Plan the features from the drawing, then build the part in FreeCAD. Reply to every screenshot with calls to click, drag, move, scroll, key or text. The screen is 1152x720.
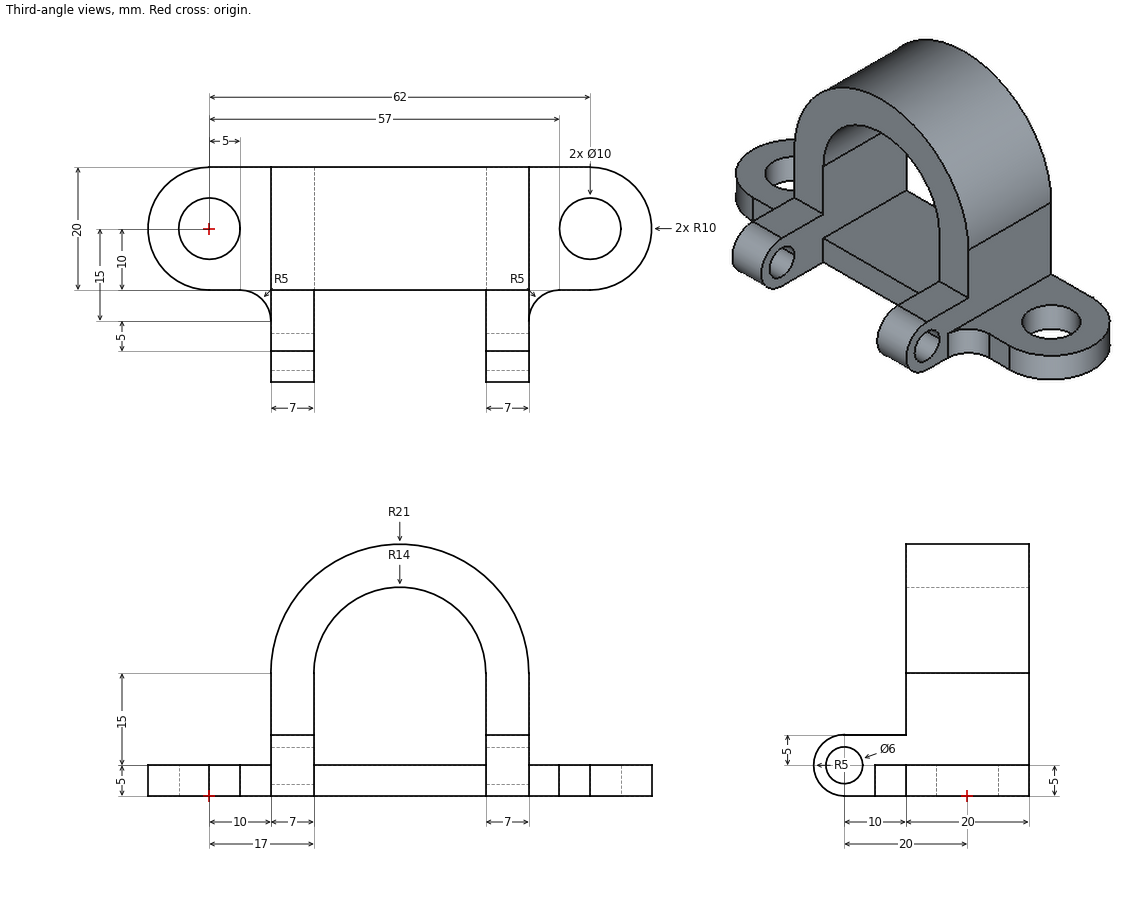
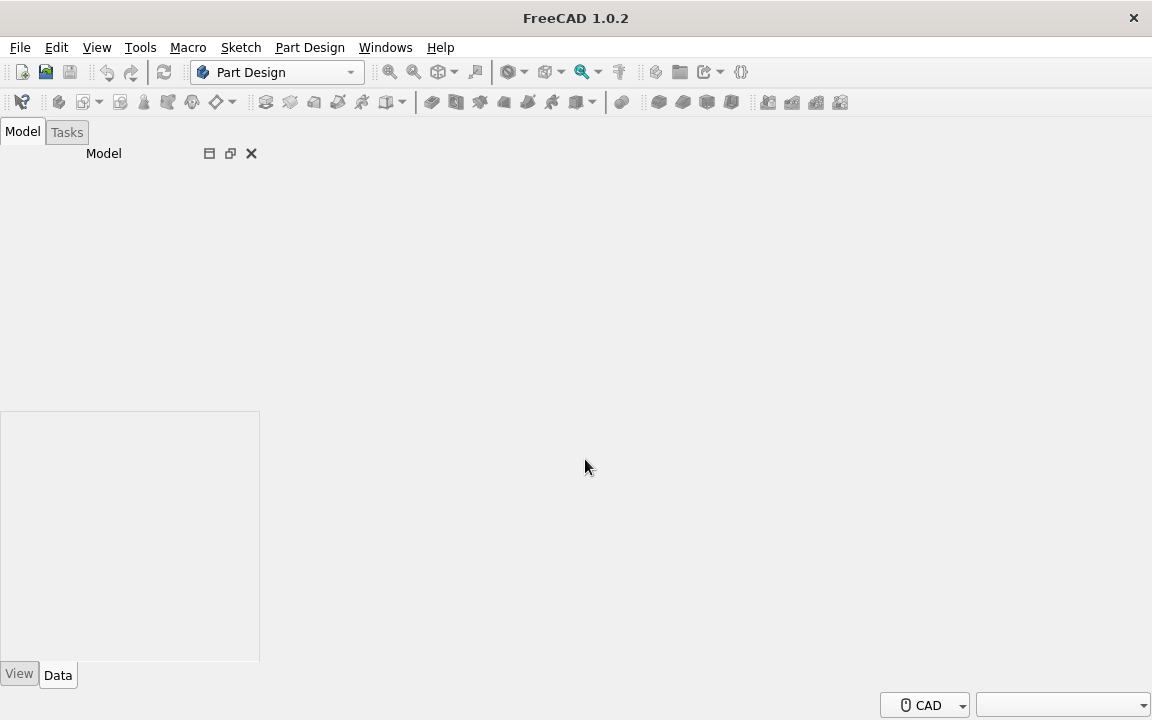
click(22, 72)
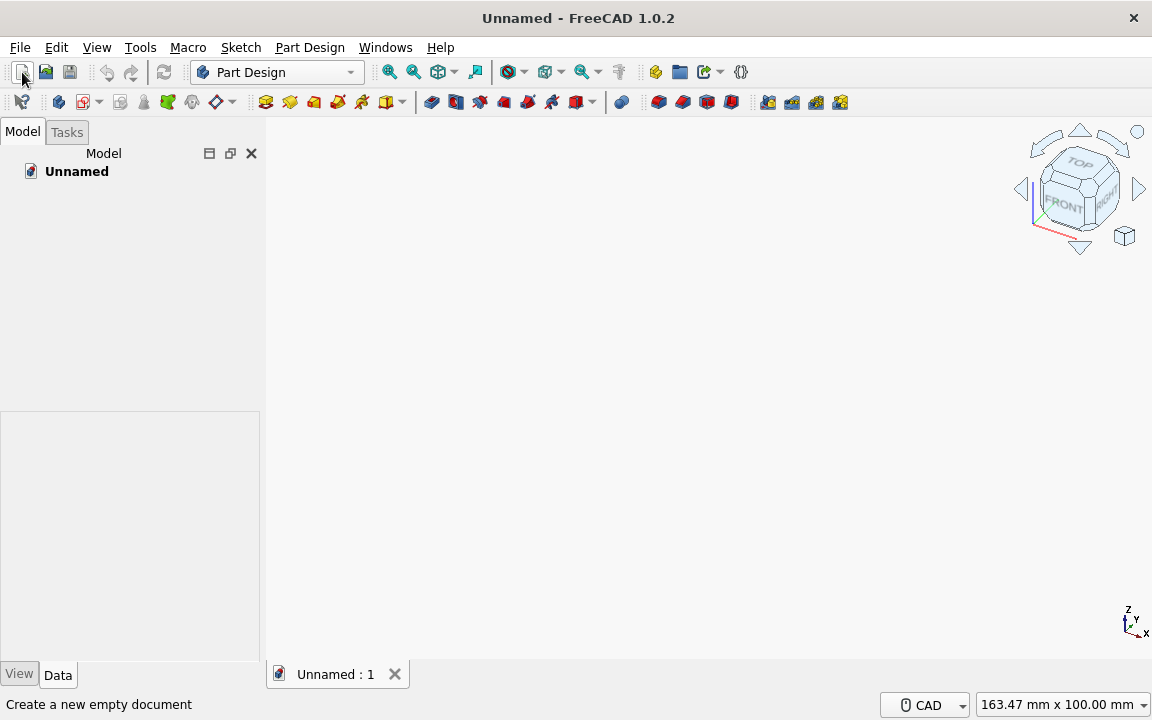
click(84, 102)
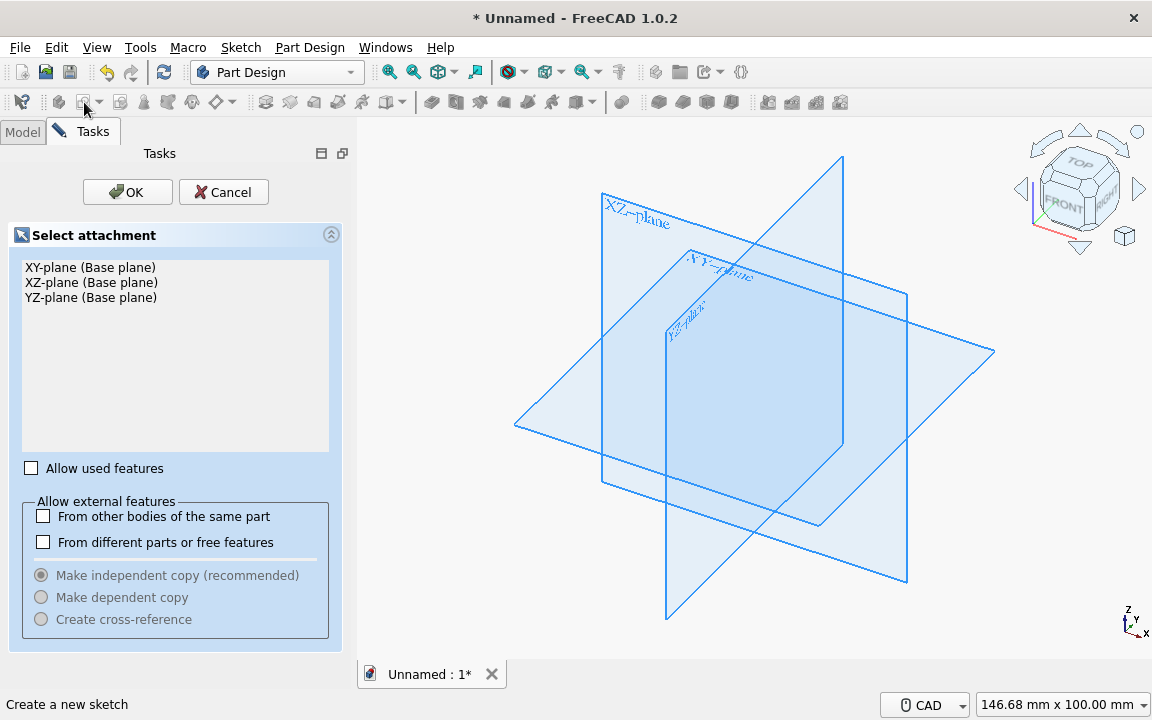
click(82, 268)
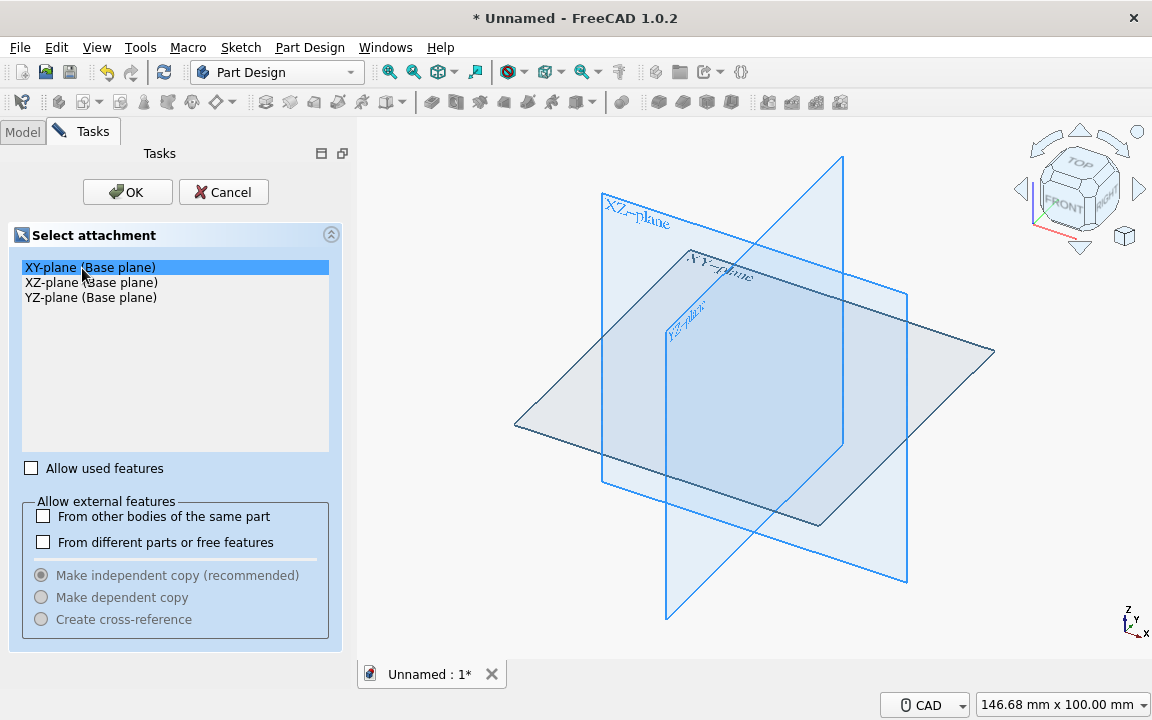
click(128, 192)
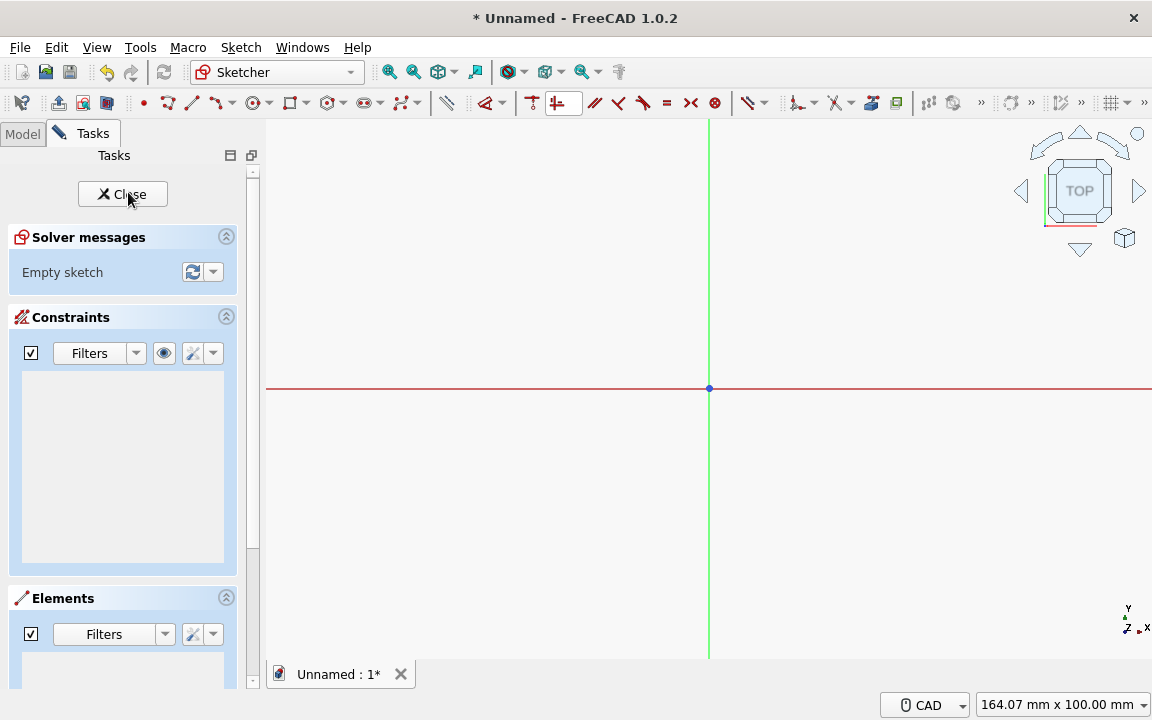
scroll(294, 389, down, 1)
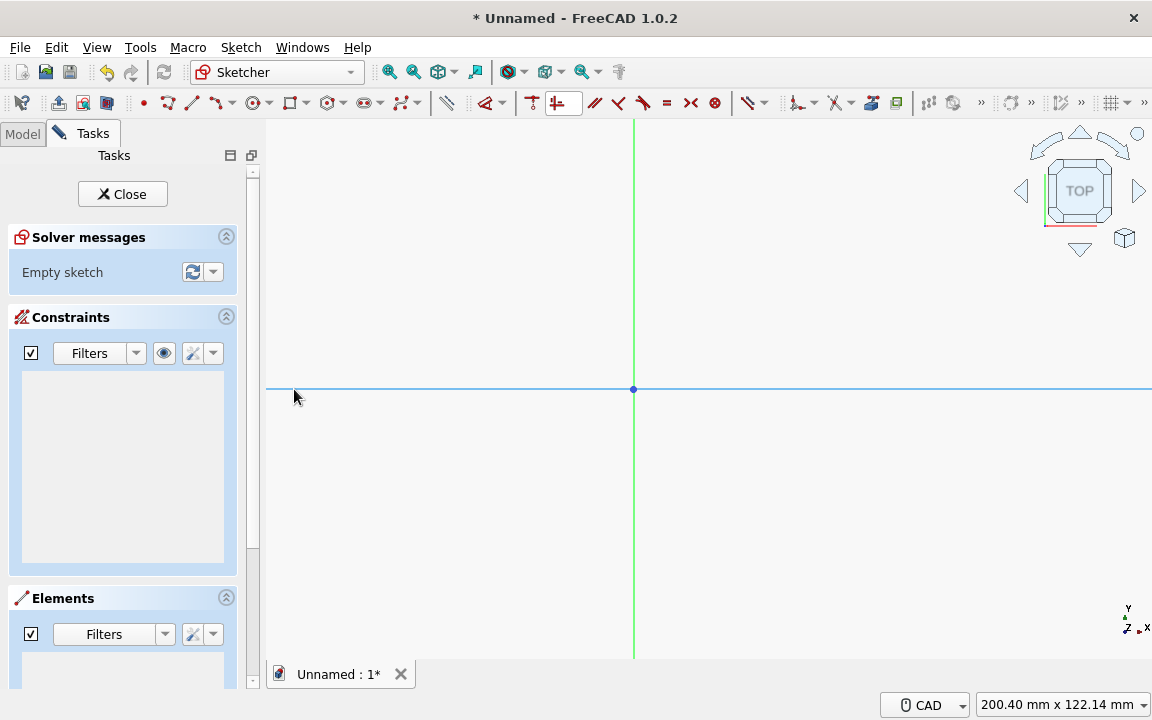
click(364, 104)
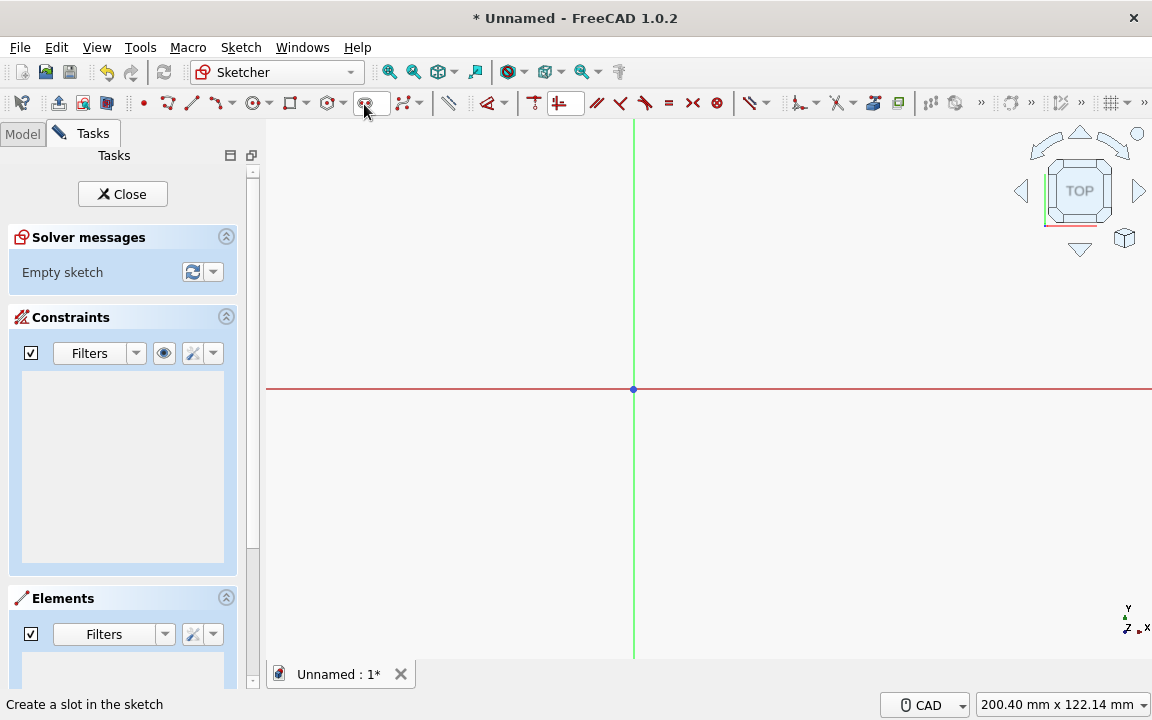
click(634, 389)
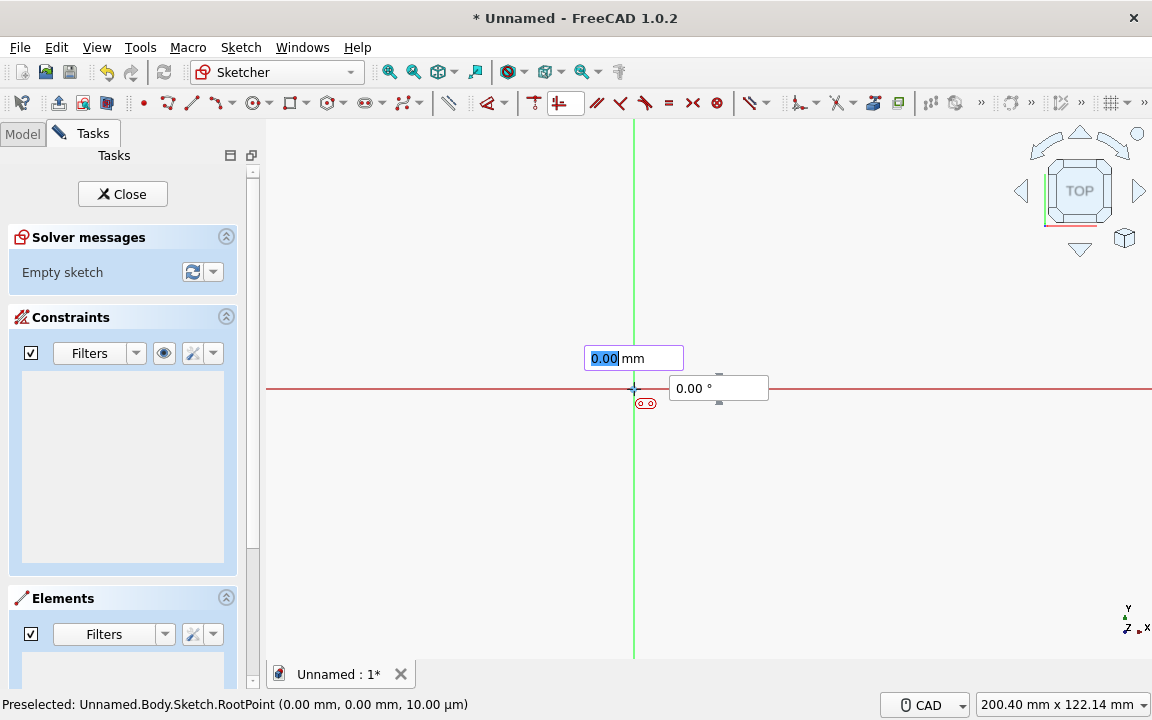
click(908, 380)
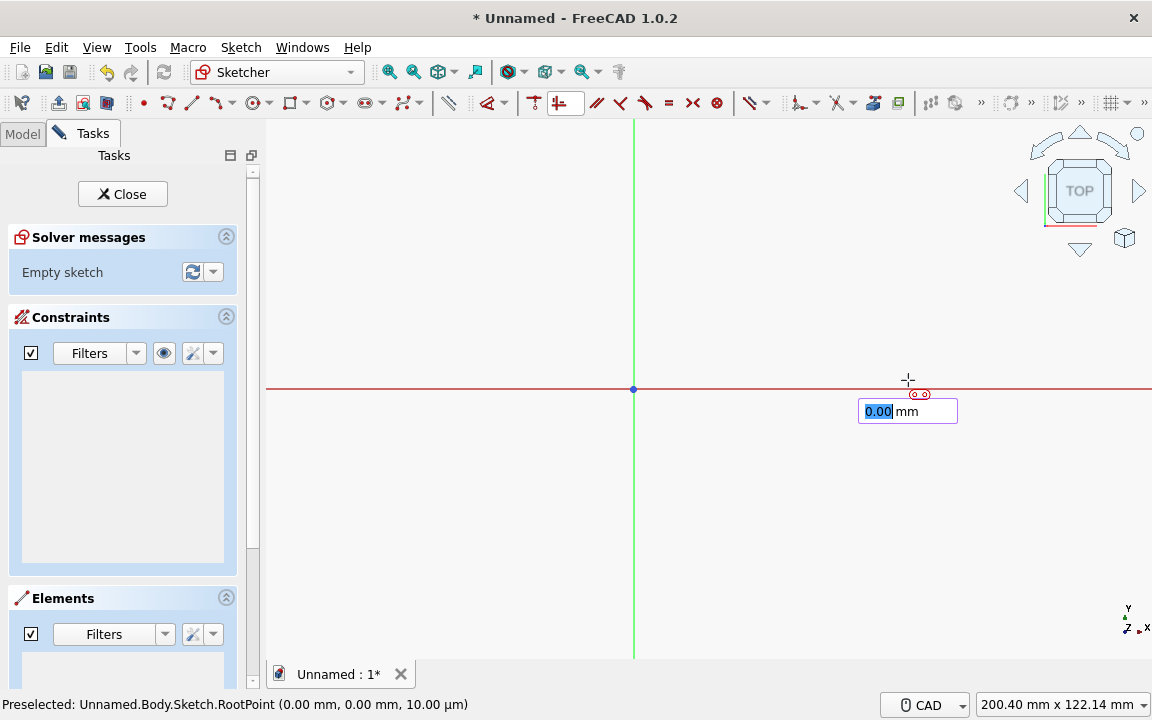
click(771, 433)
key(Escape)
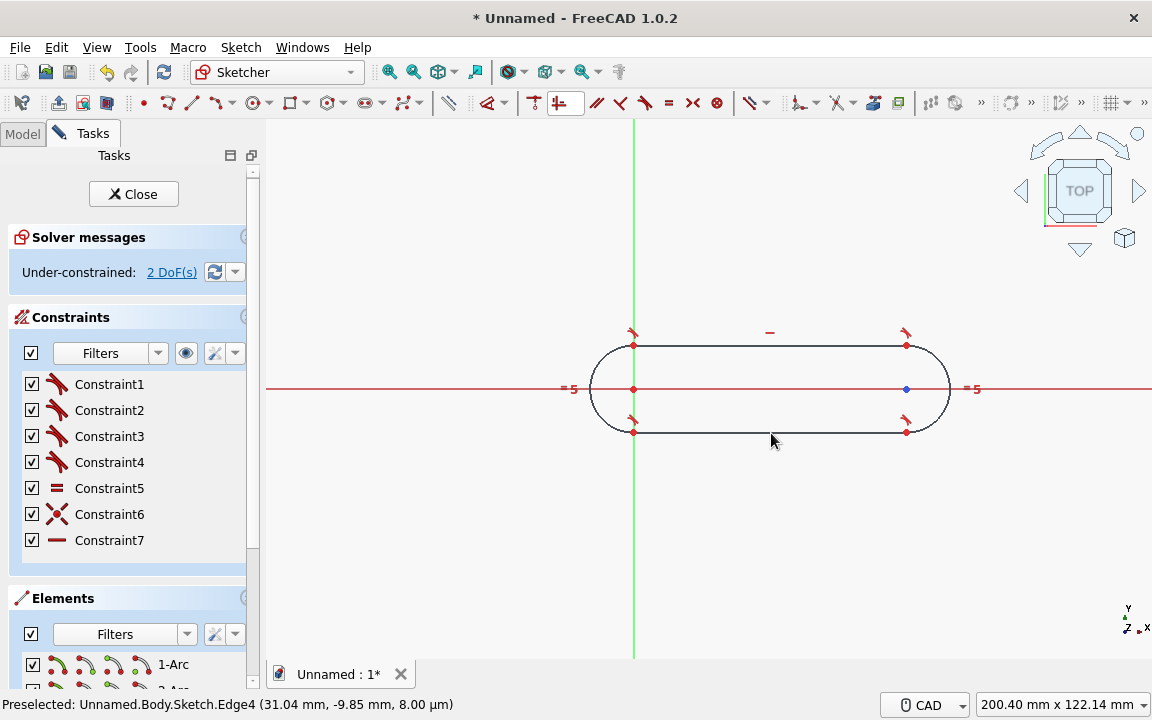
click(488, 104)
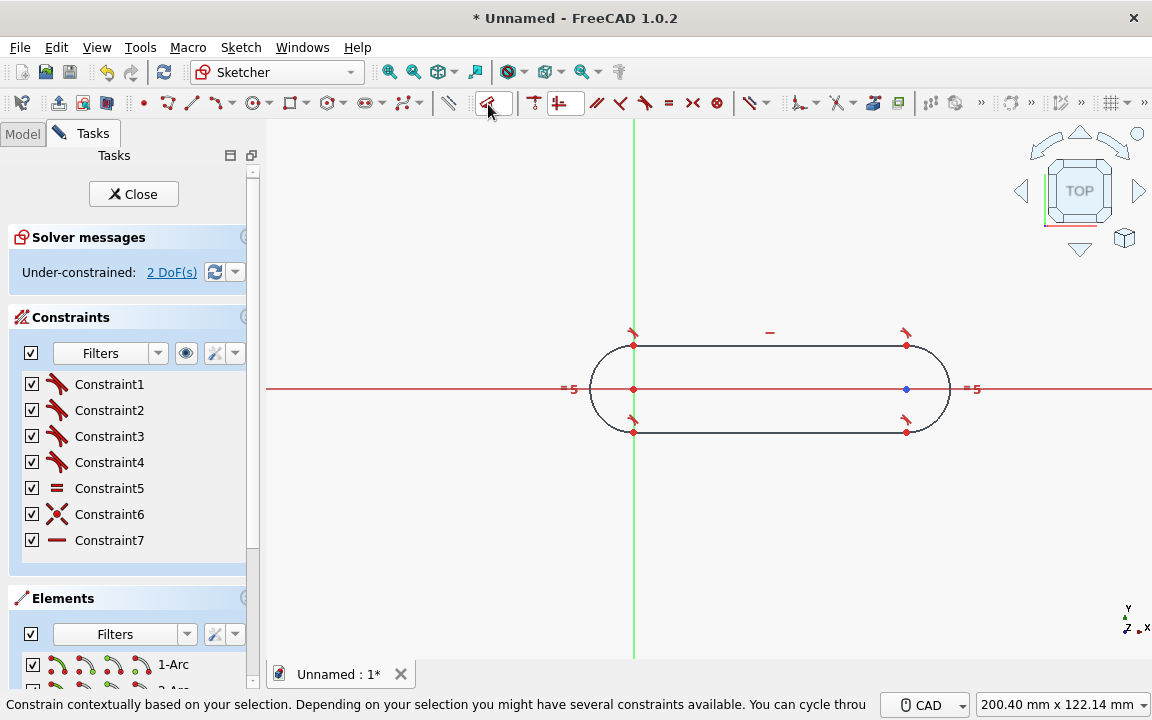
click(599, 363)
click(573, 344)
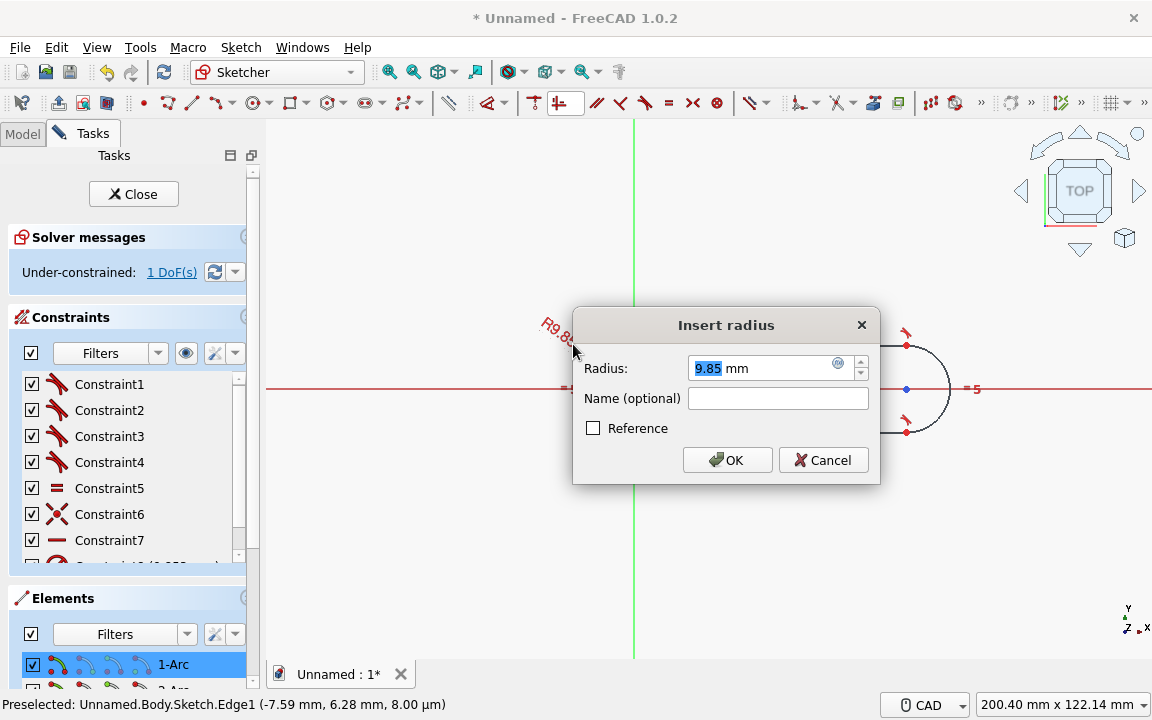
text(10)
key(Return)